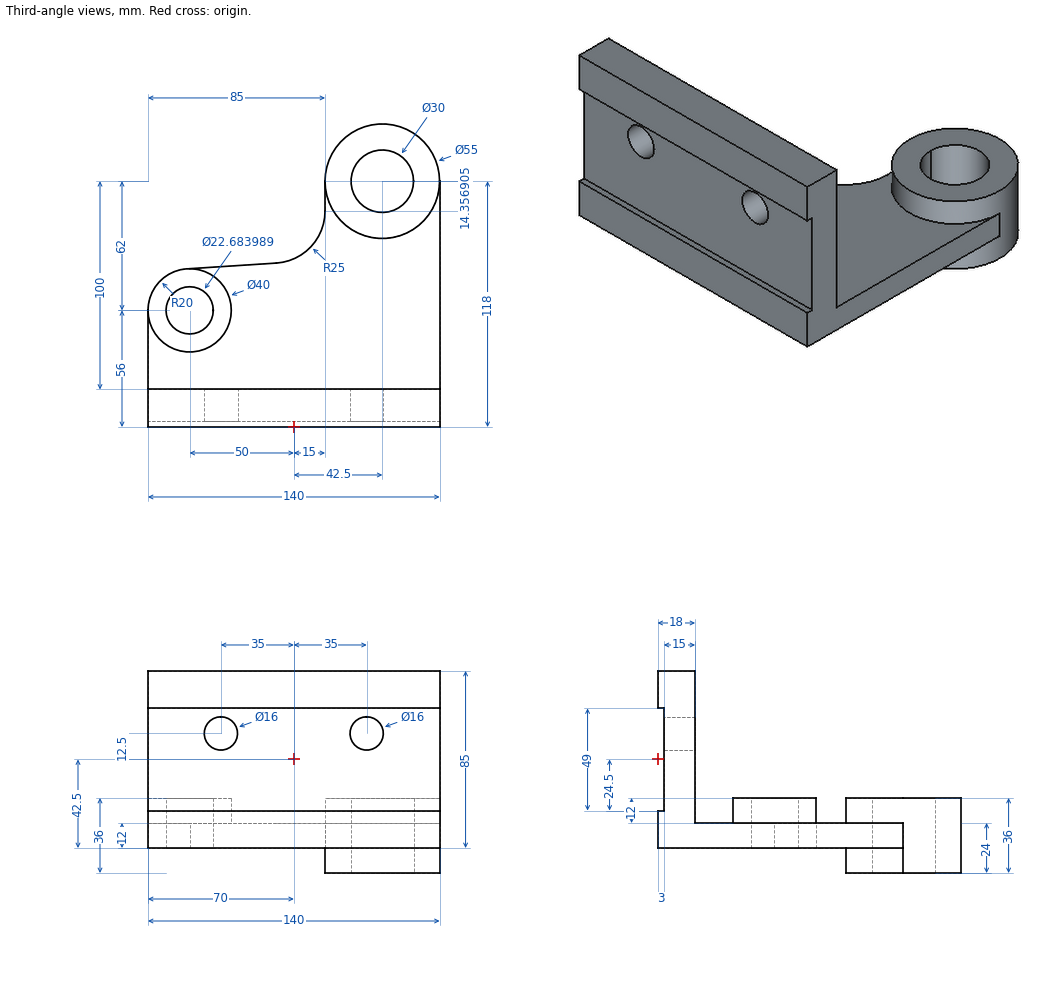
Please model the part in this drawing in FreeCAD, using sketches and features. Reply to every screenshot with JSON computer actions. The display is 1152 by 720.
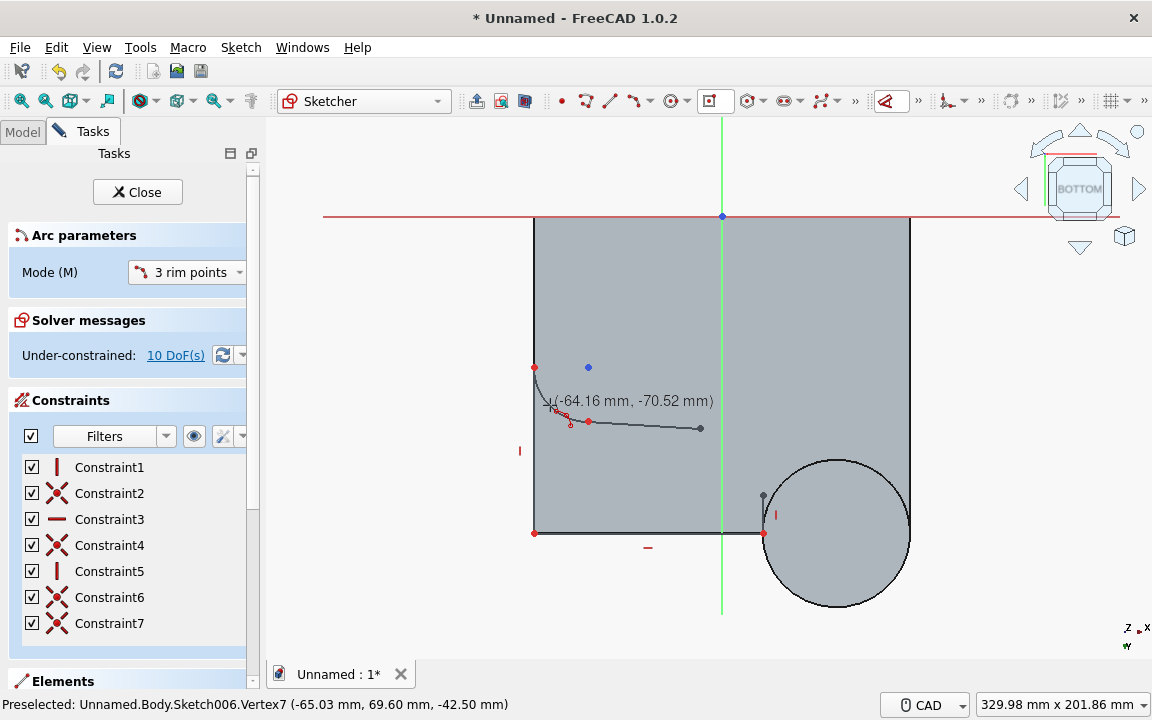
{"action": "left_click", "coordinate": [700, 429]}
{"action": "left_click", "coordinate": [763, 496]}
{"action": "left_click", "coordinate": [744, 449]}
{"action": "key", "text": "Escape"}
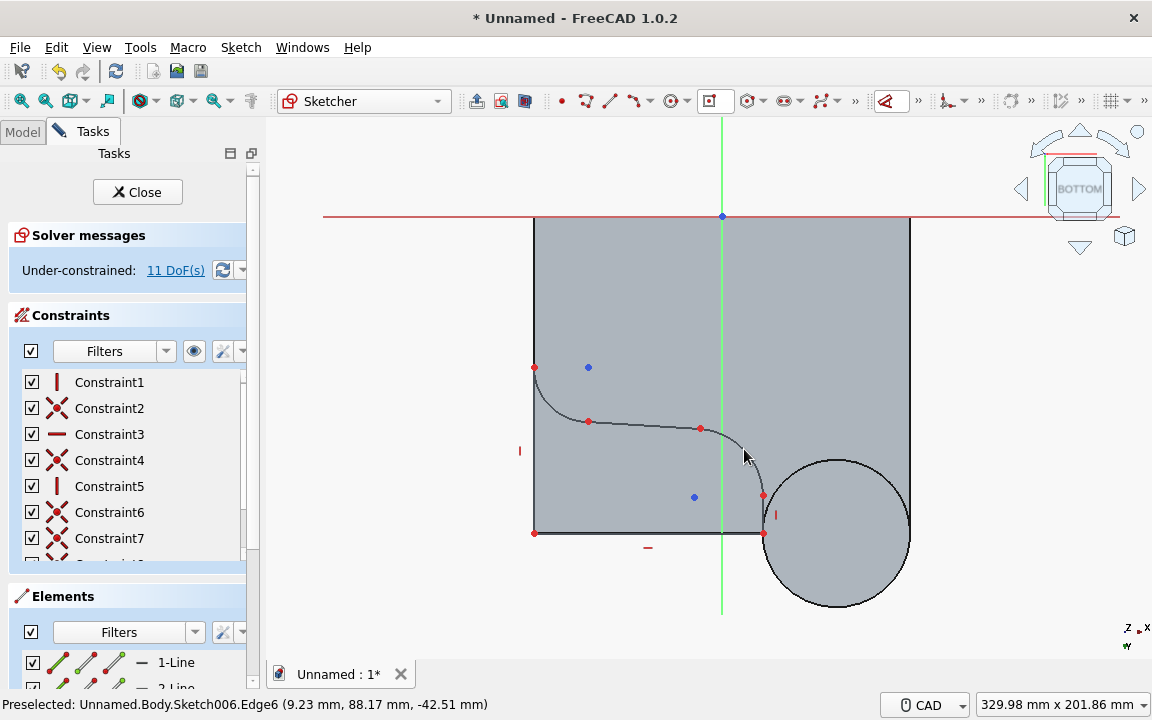
{"action": "left_click", "coordinate": [763, 507]}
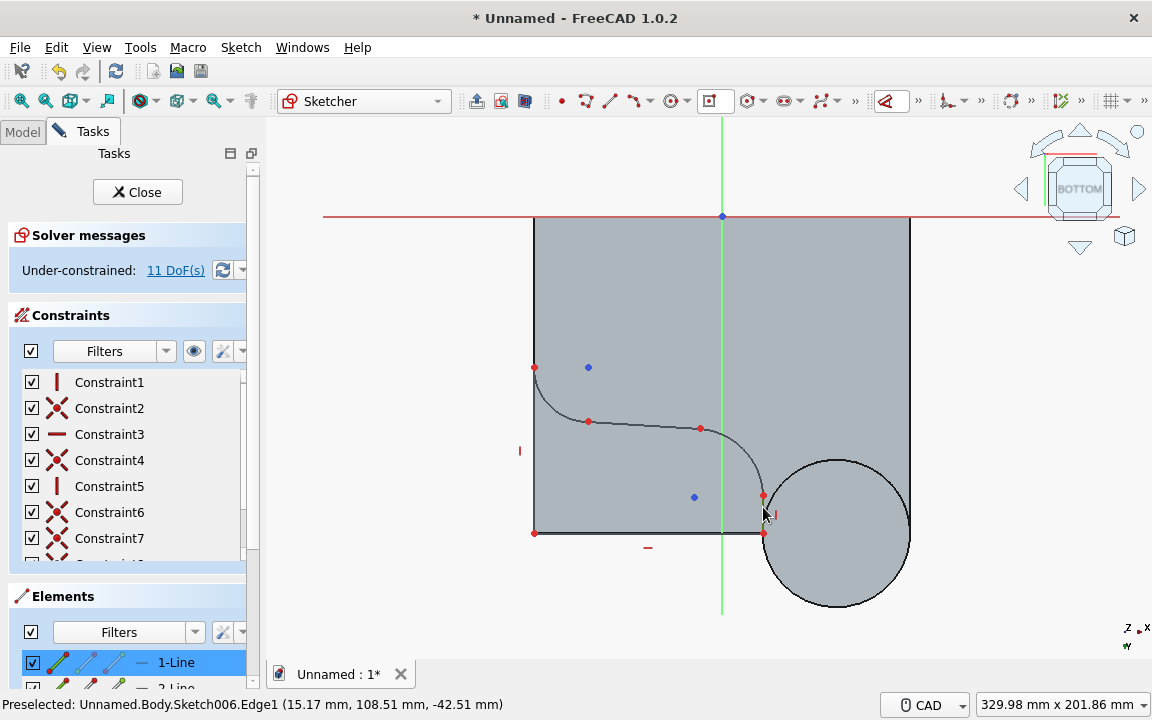
{"action": "left_click", "coordinate": [756, 467]}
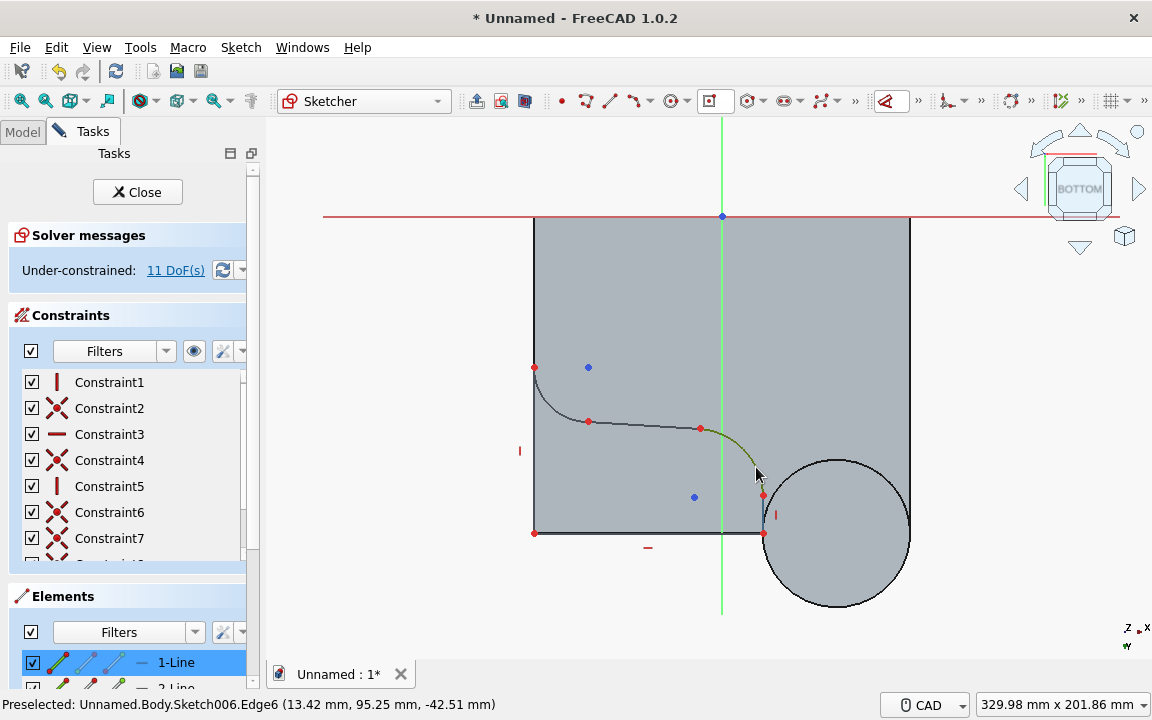
{"action": "key", "text": "t"}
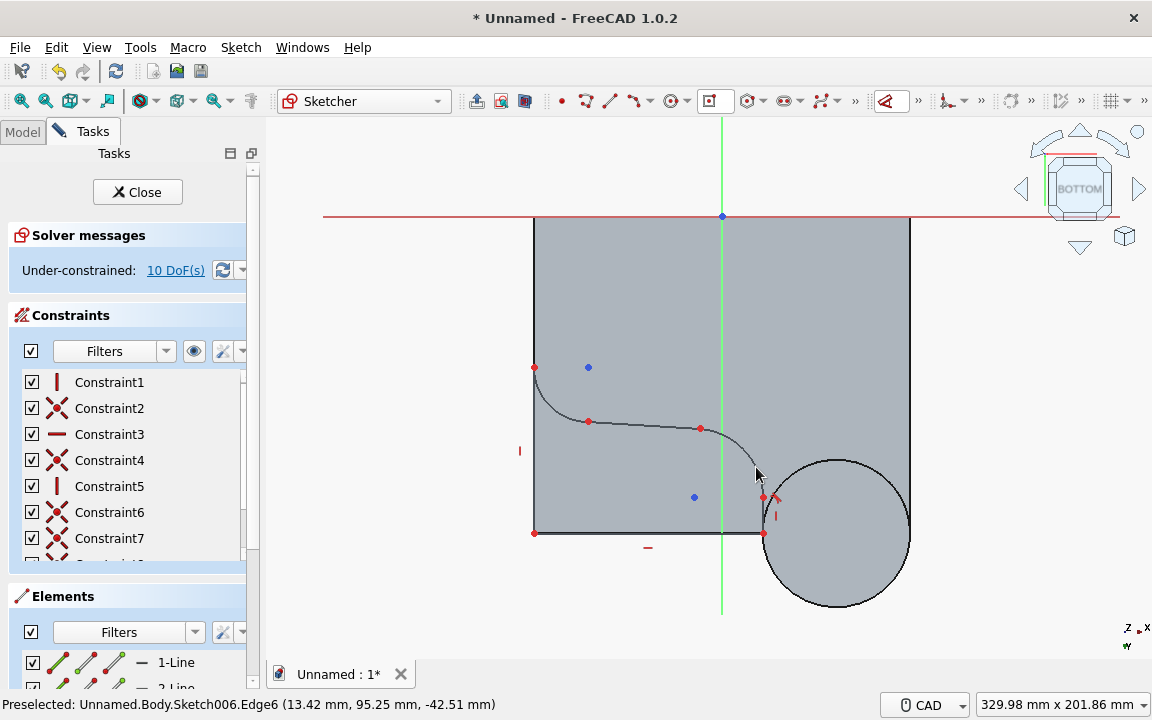
{"action": "left_click", "coordinate": [534, 484]}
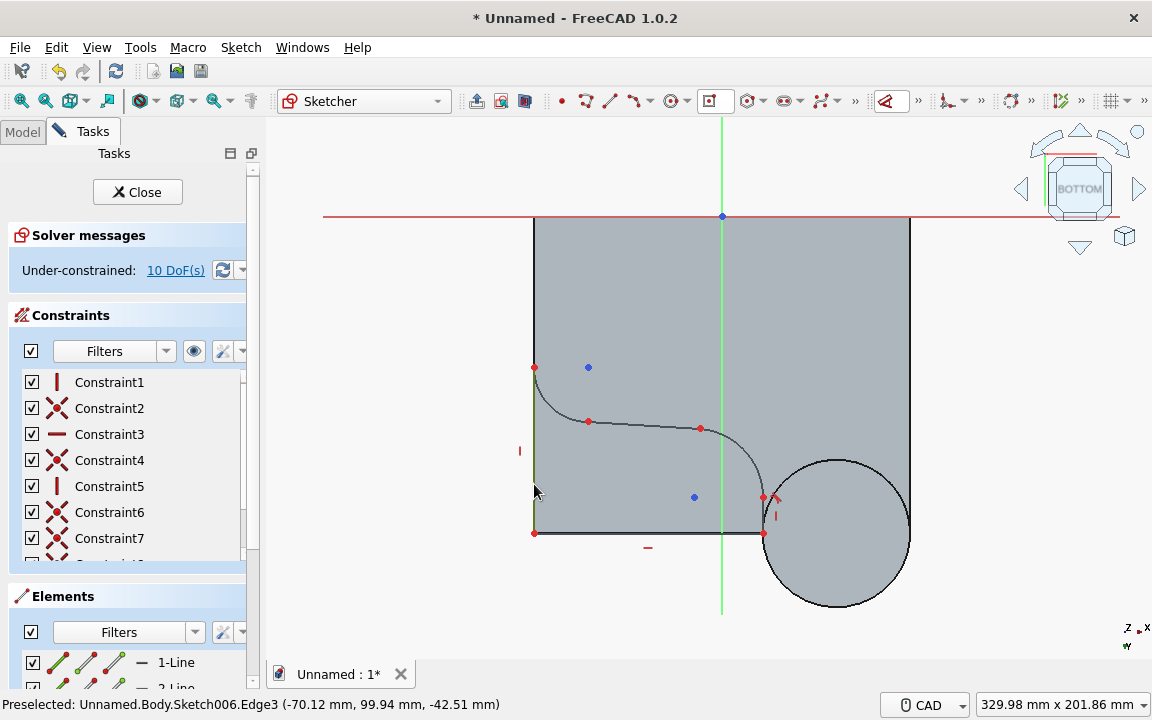
{"action": "left_click", "coordinate": [564, 416]}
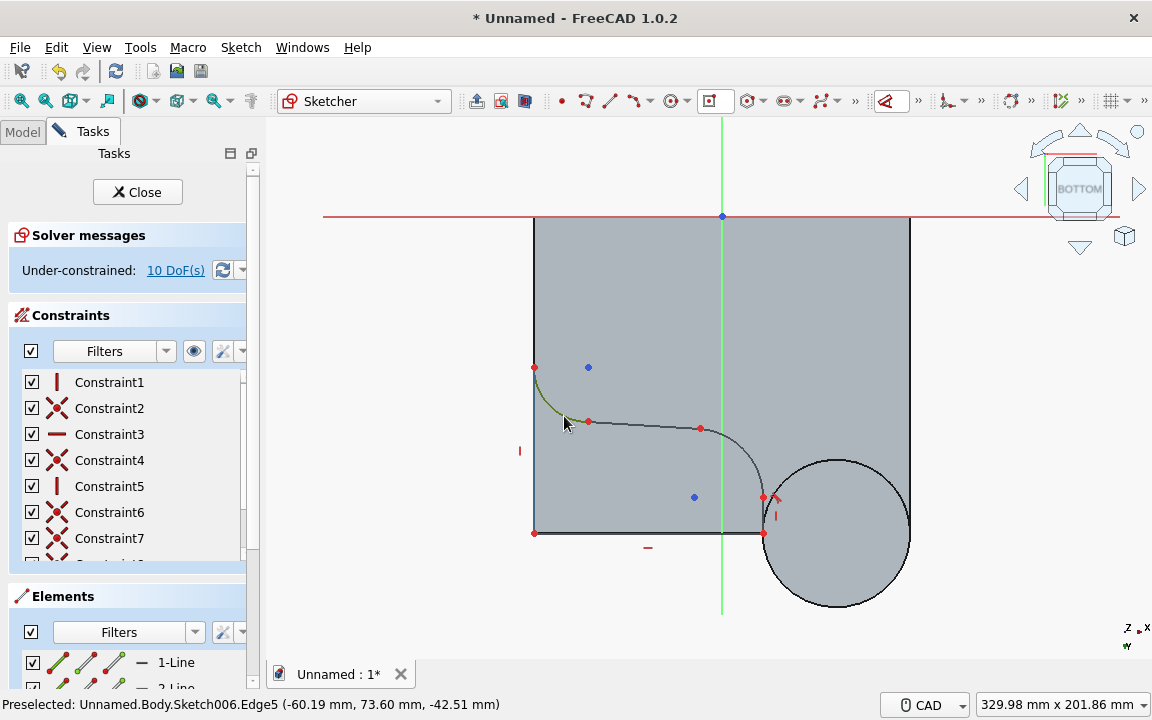
{"action": "key", "text": "t"}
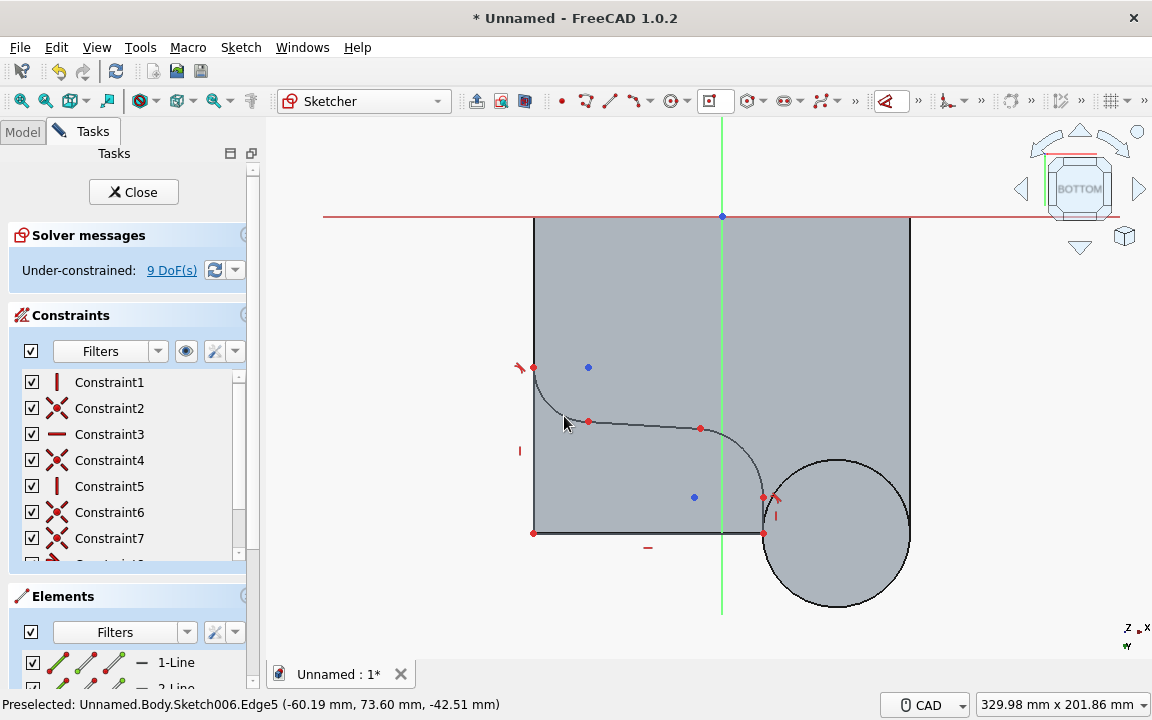
{"action": "left_click", "coordinate": [622, 424]}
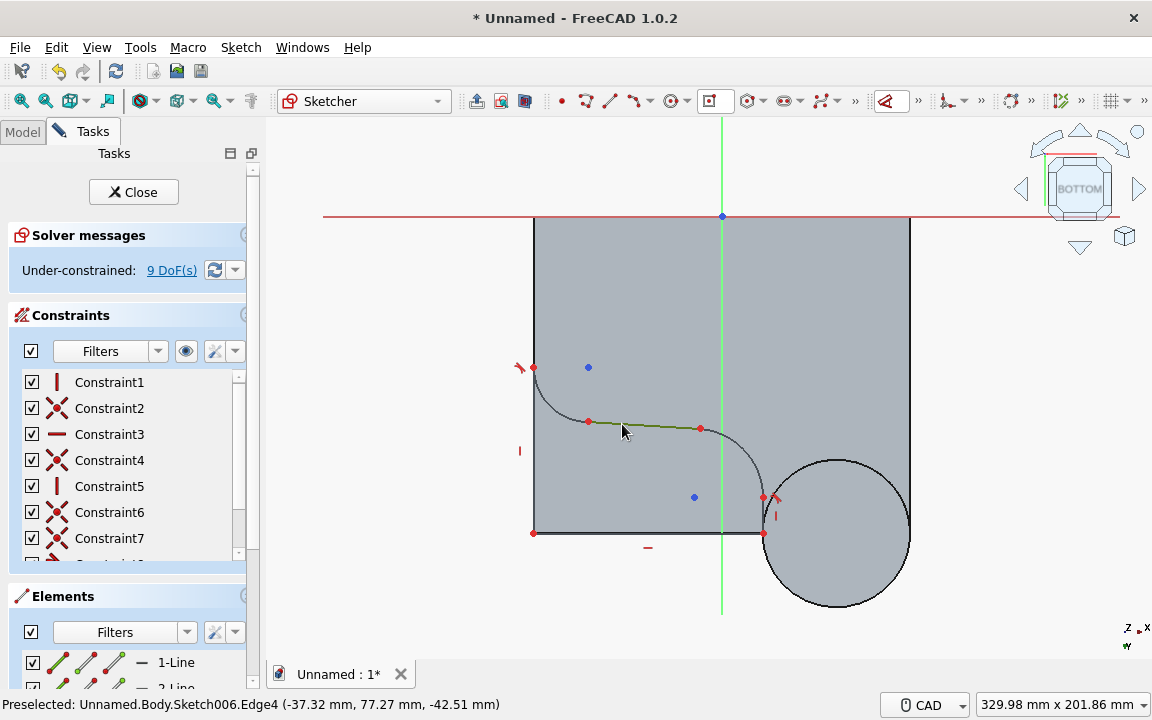
{"action": "left_click", "coordinate": [756, 468]}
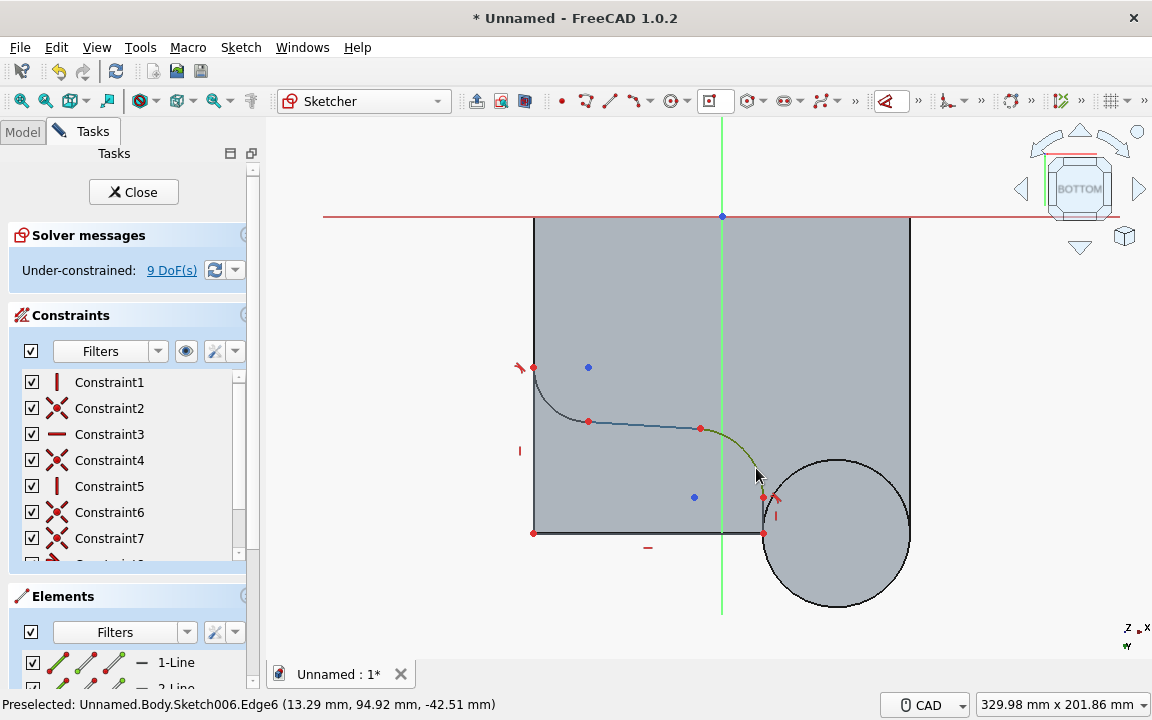
{"action": "key", "text": "t"}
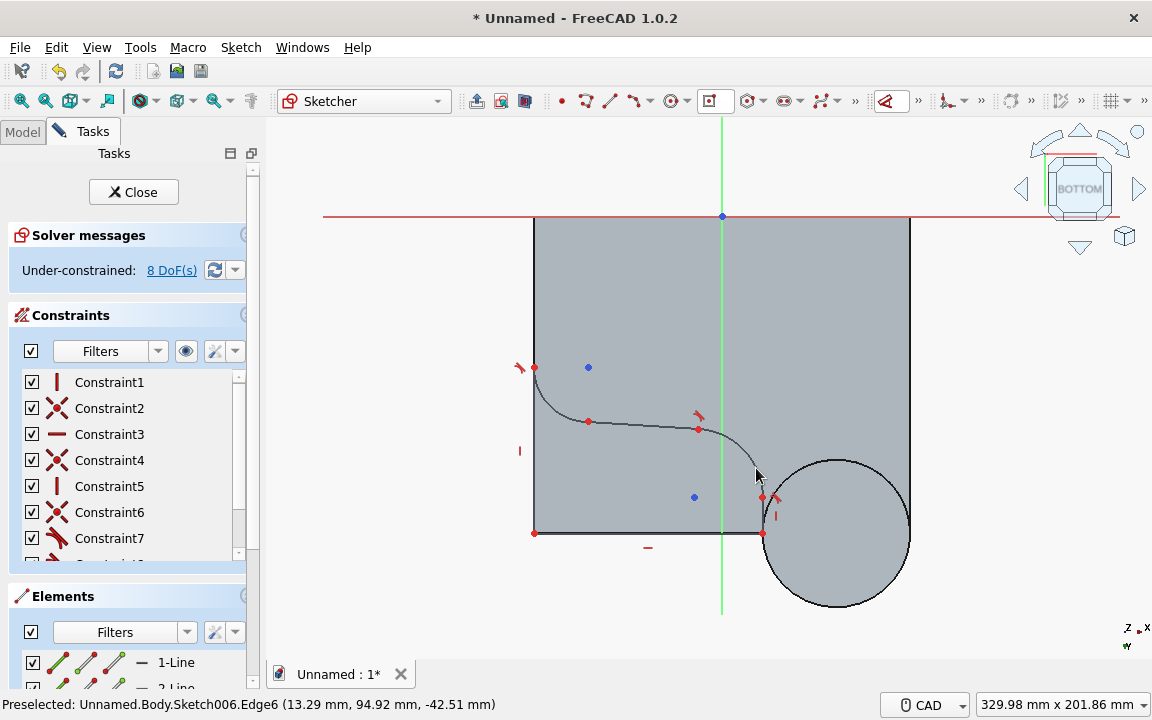
{"action": "left_click", "coordinate": [563, 416]}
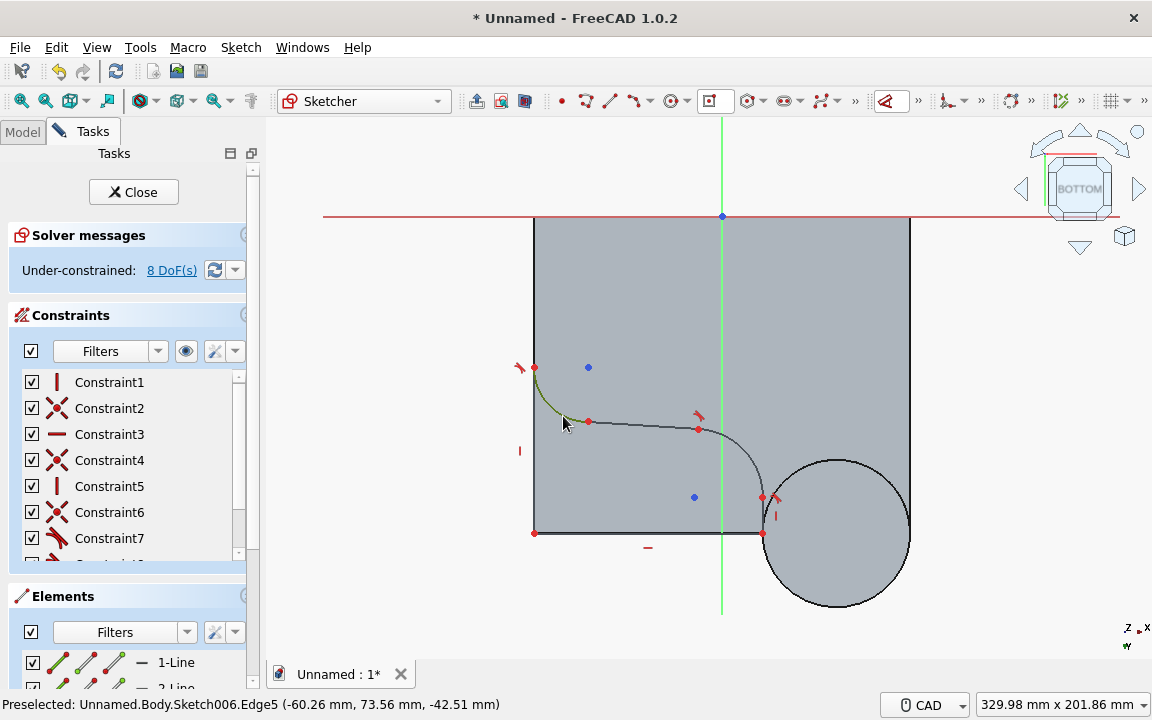
{"action": "key", "text": "k r"}